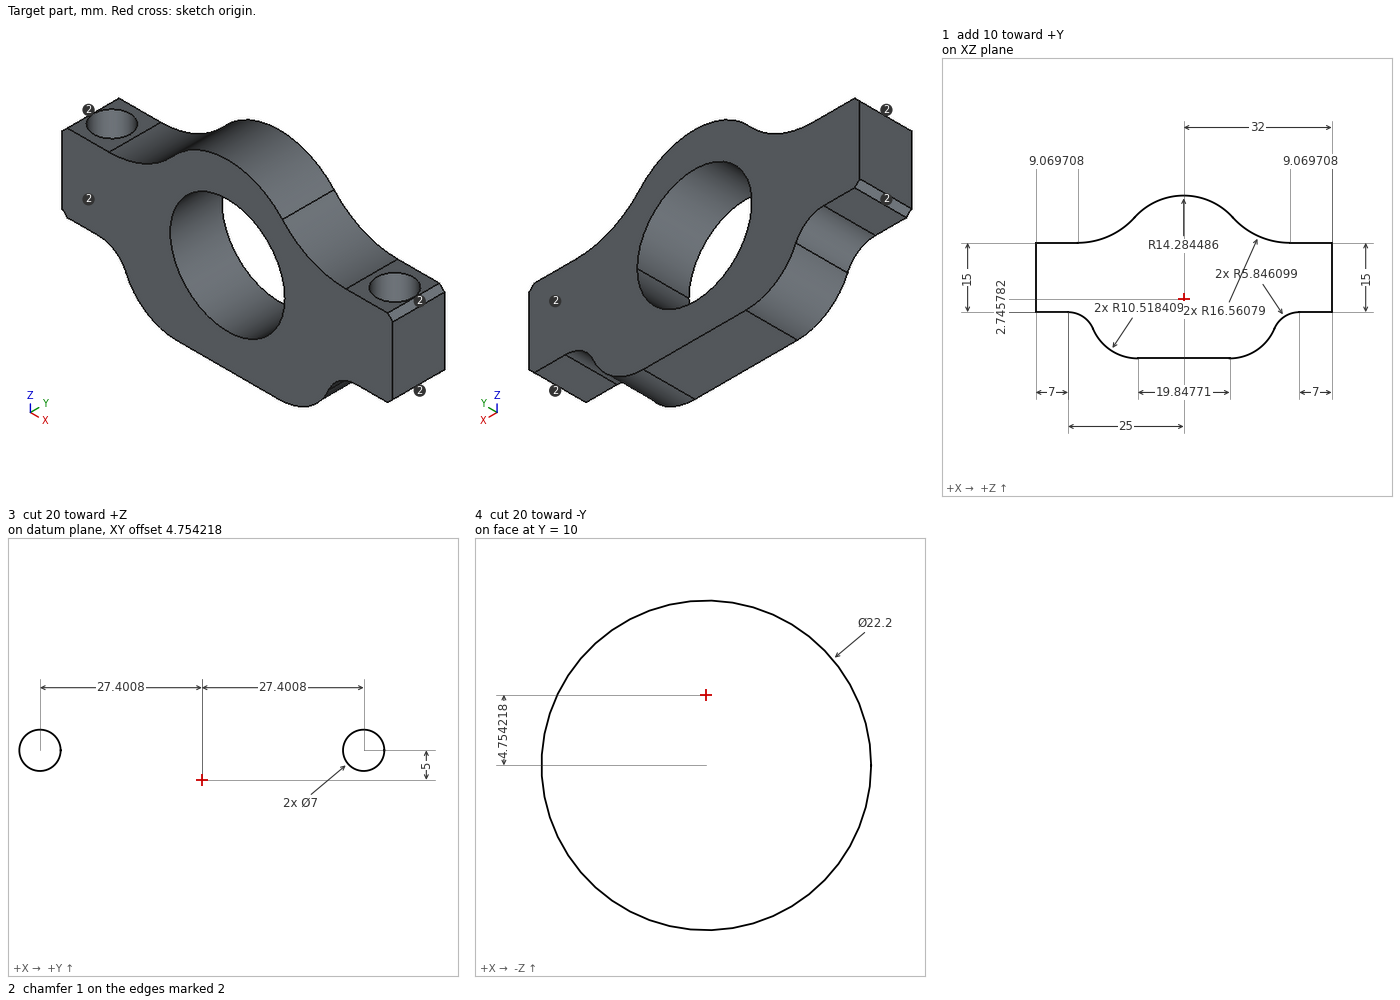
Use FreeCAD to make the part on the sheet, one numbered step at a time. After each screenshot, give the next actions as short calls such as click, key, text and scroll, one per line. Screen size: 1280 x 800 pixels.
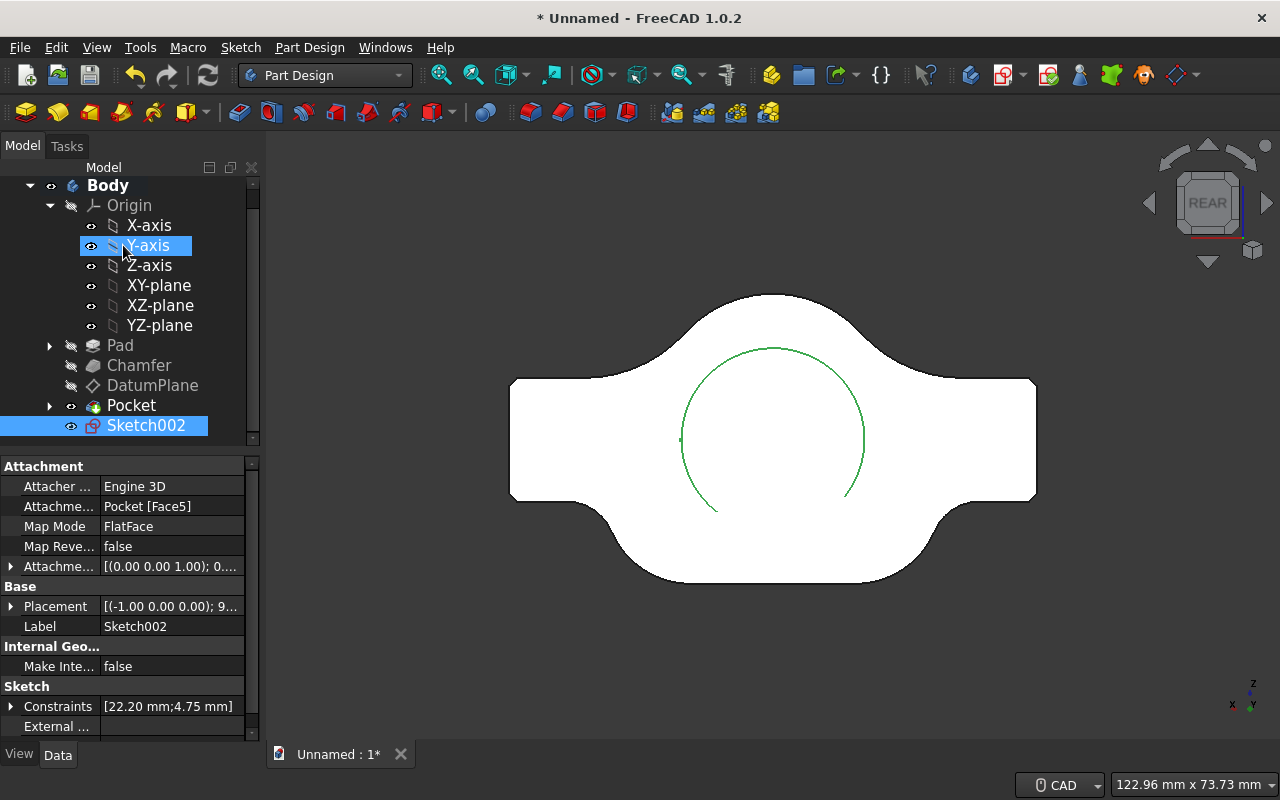
click(240, 112)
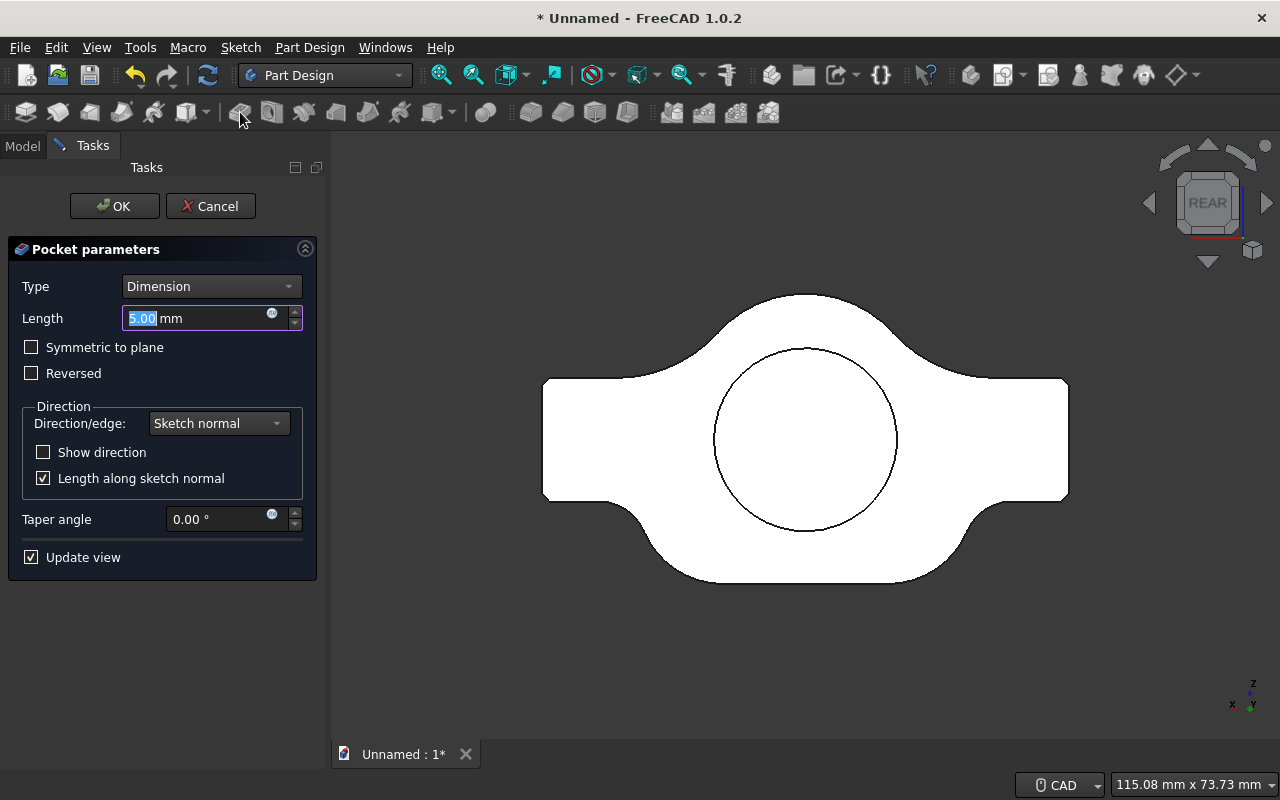
text(20)
key(Tab)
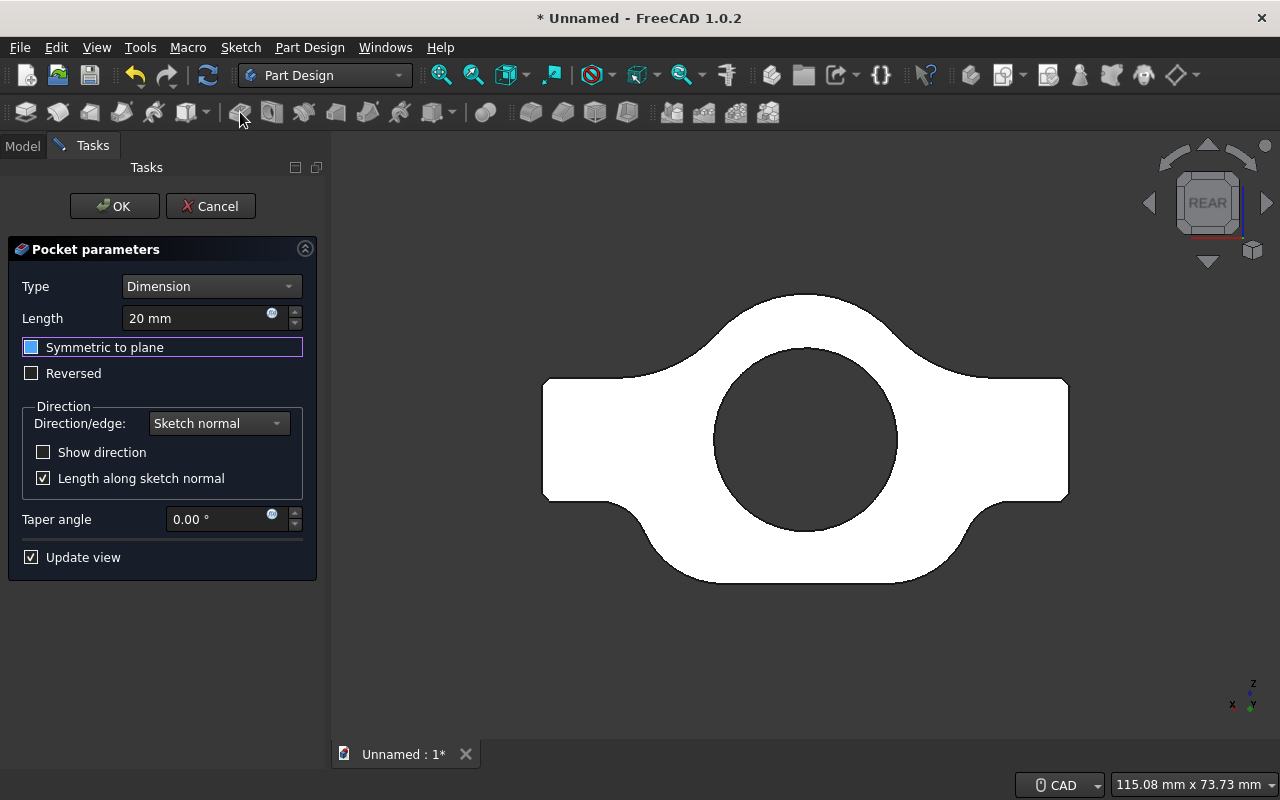
click(115, 206)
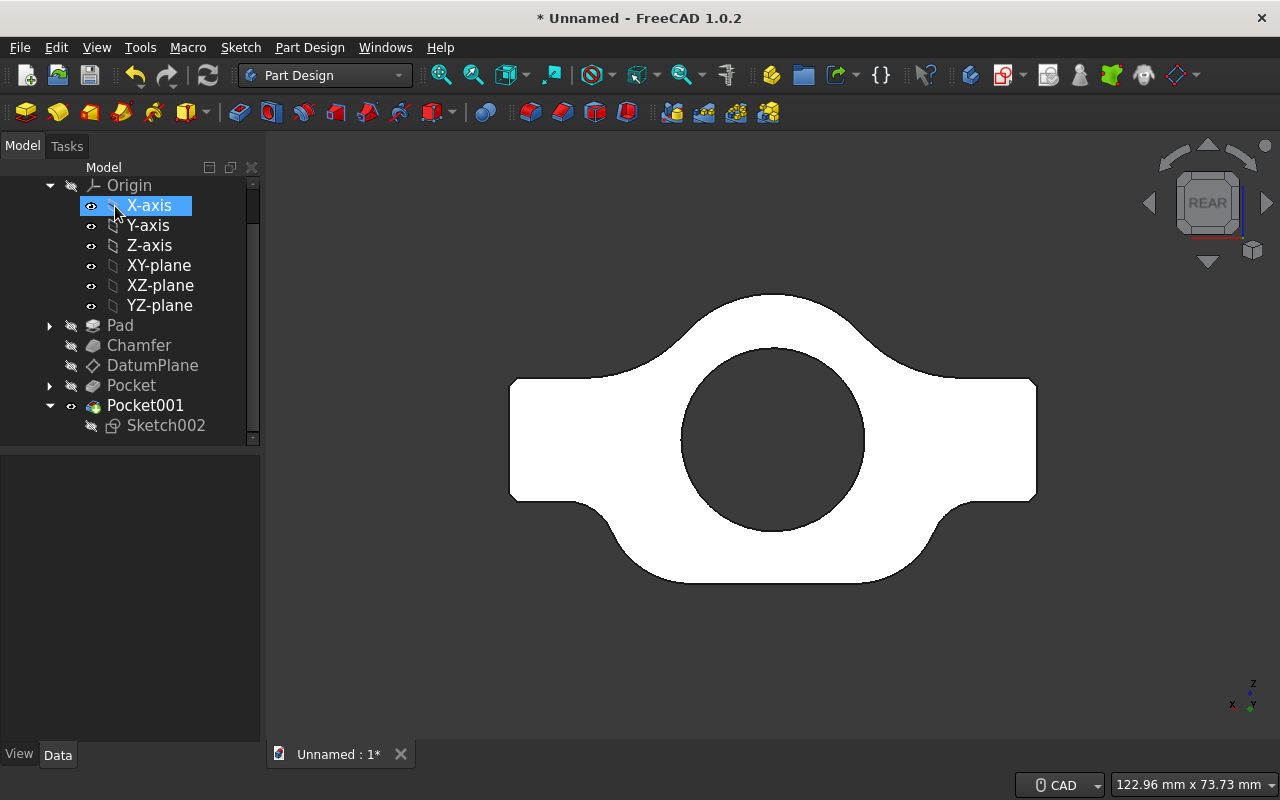
key(0)